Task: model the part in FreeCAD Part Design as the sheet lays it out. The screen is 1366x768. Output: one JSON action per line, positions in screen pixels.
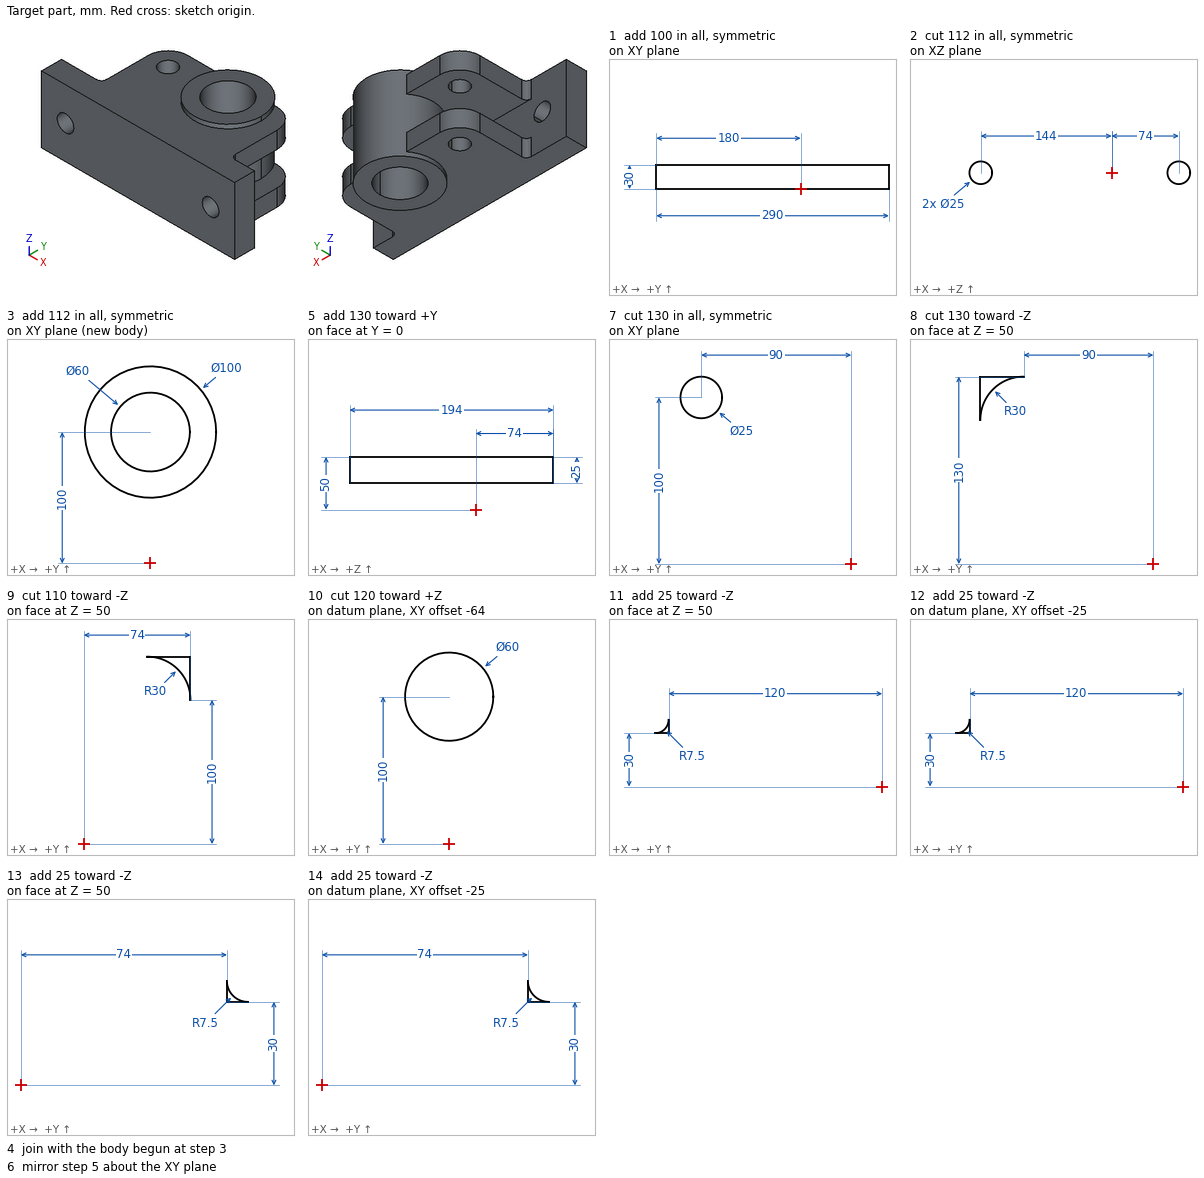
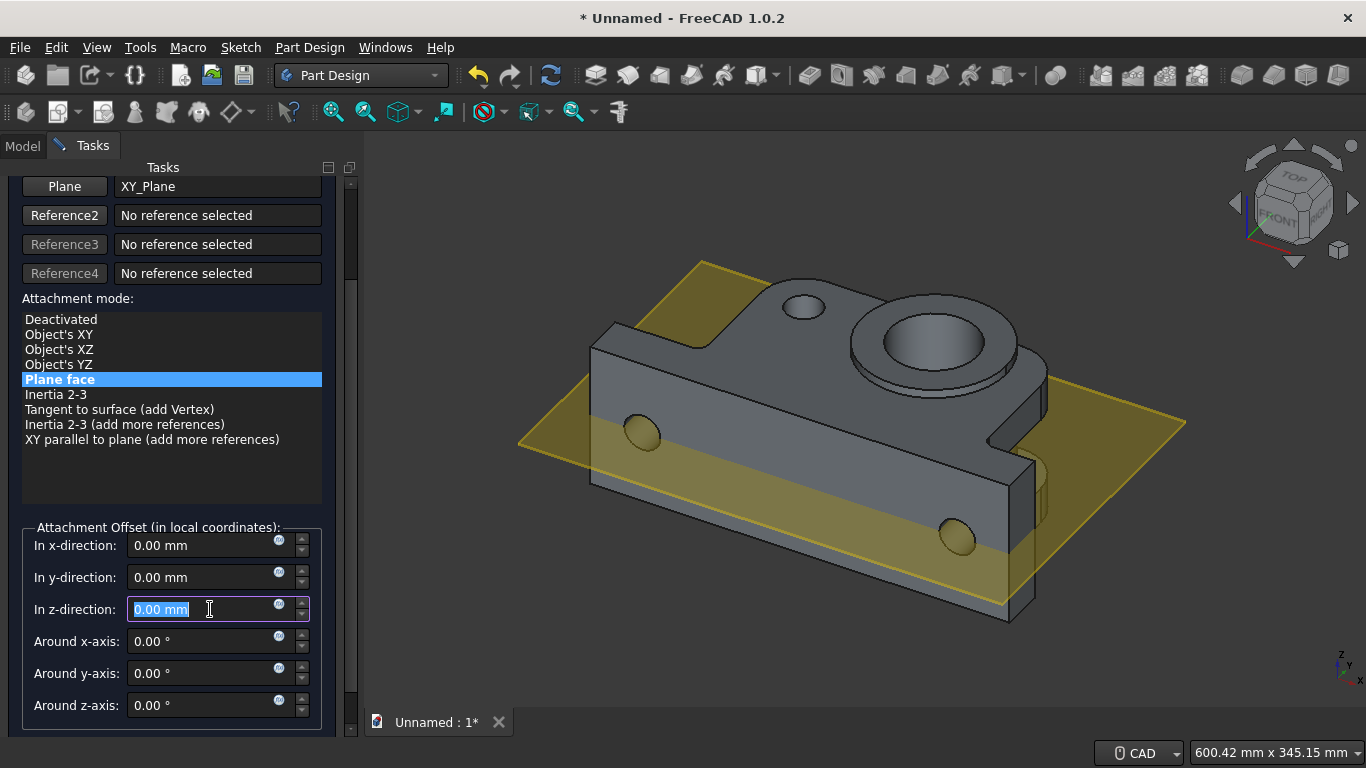
{"action": "type", "text": "-25"}
{"action": "key", "text": "Tab"}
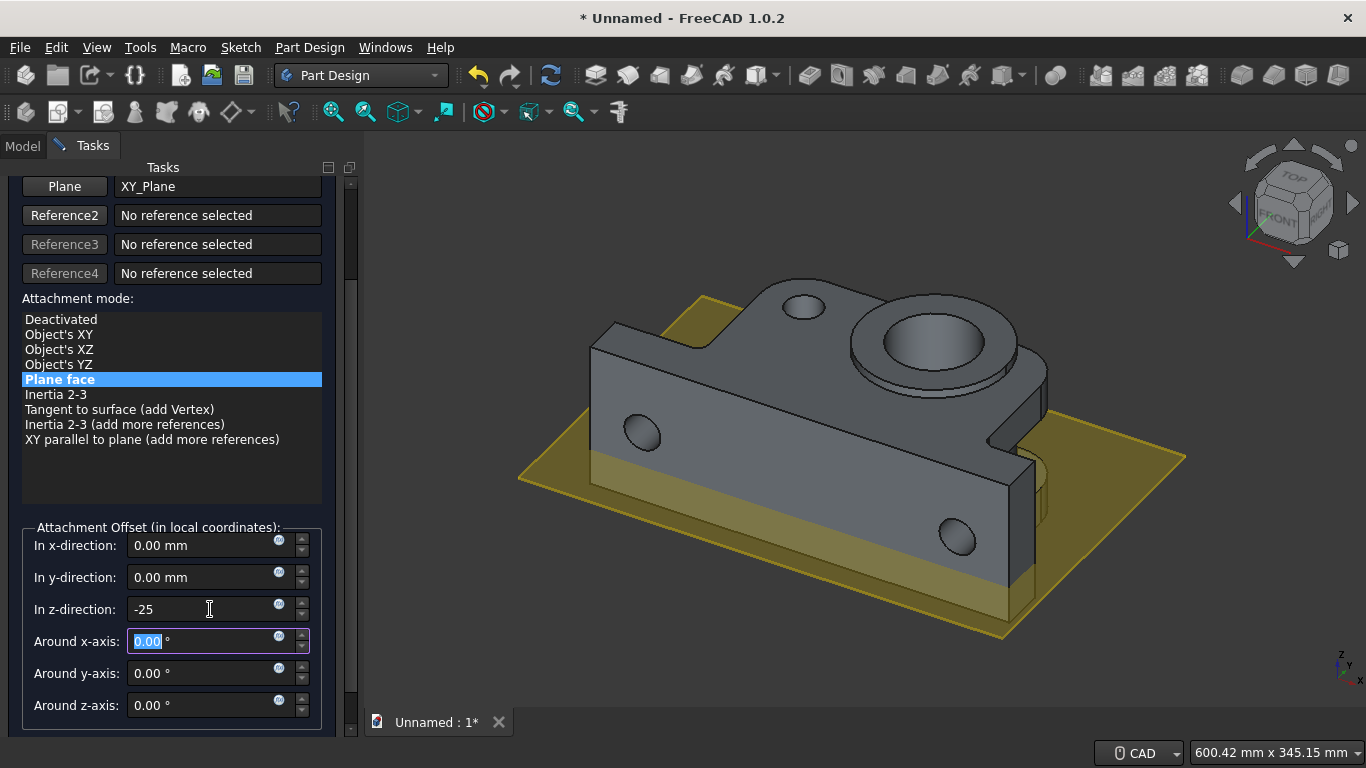
{"action": "scroll", "coordinate": [351, 456], "scroll_direction": "up", "scroll_amount": 3}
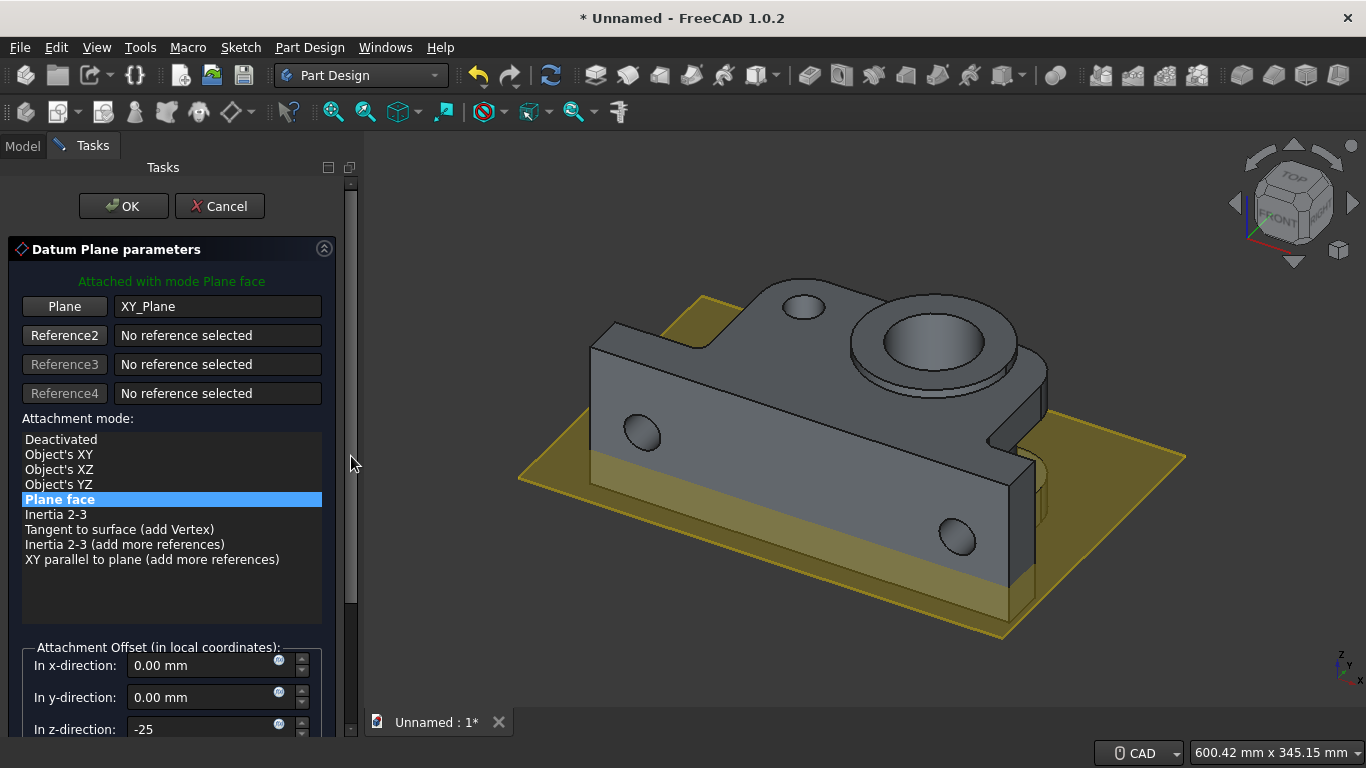
{"action": "left_click", "coordinate": [124, 206]}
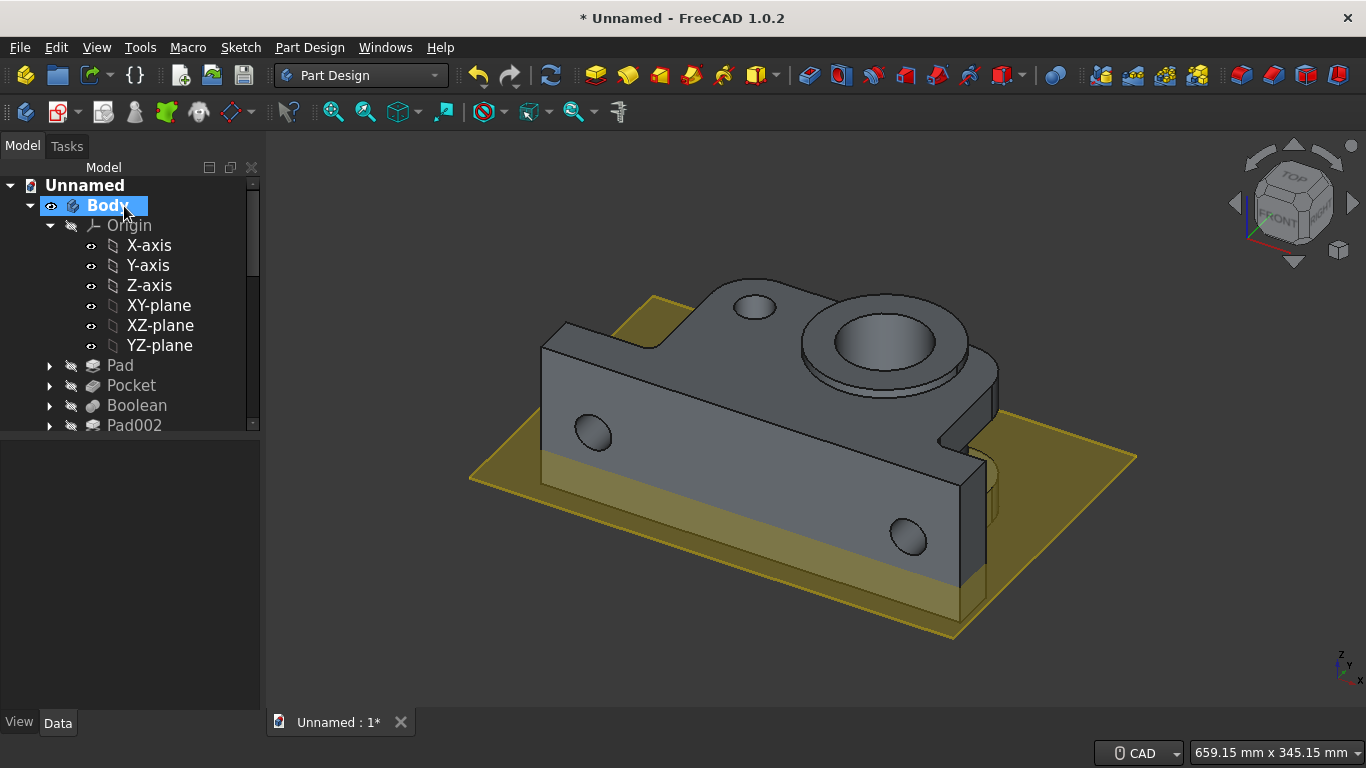
{"action": "scroll", "coordinate": [100, 301], "scroll_direction": "down", "scroll_amount": 3}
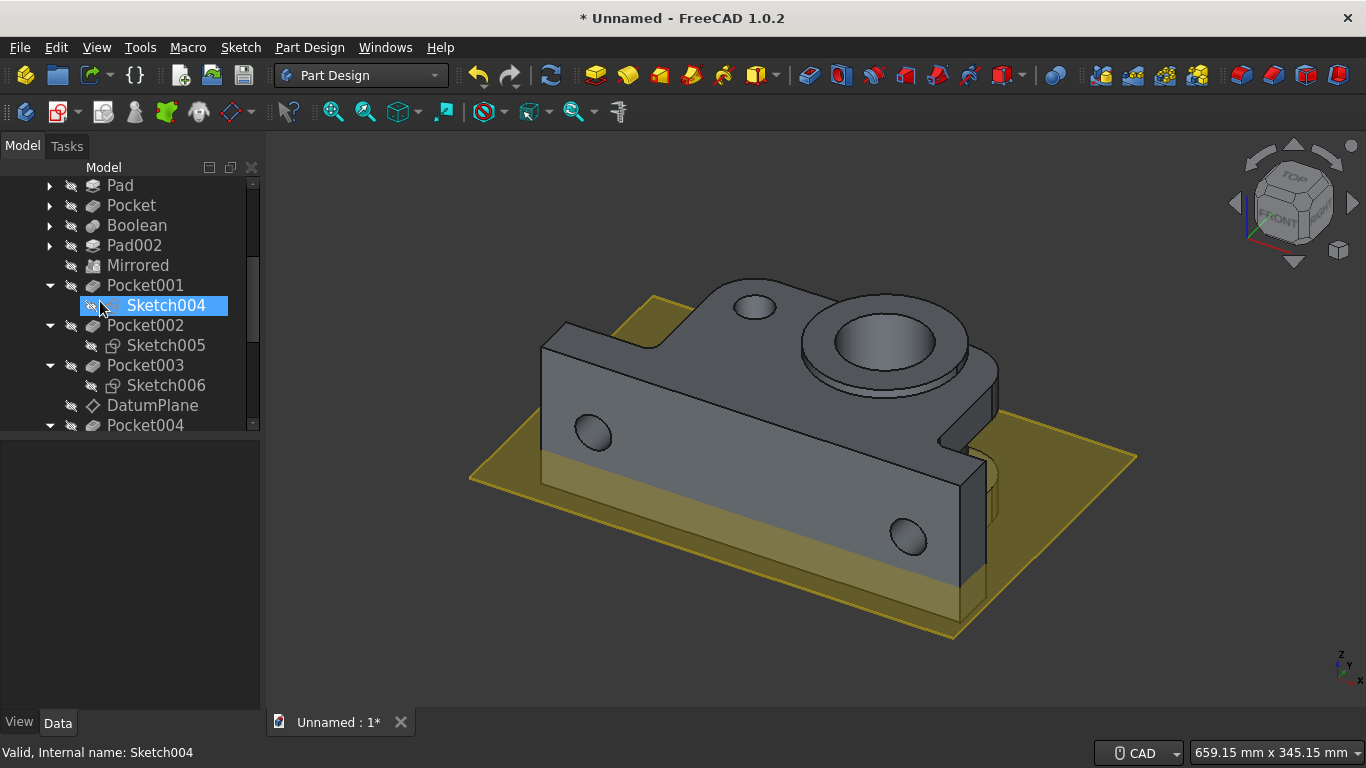
{"action": "scroll", "coordinate": [140, 301], "scroll_direction": "up", "scroll_amount": 15}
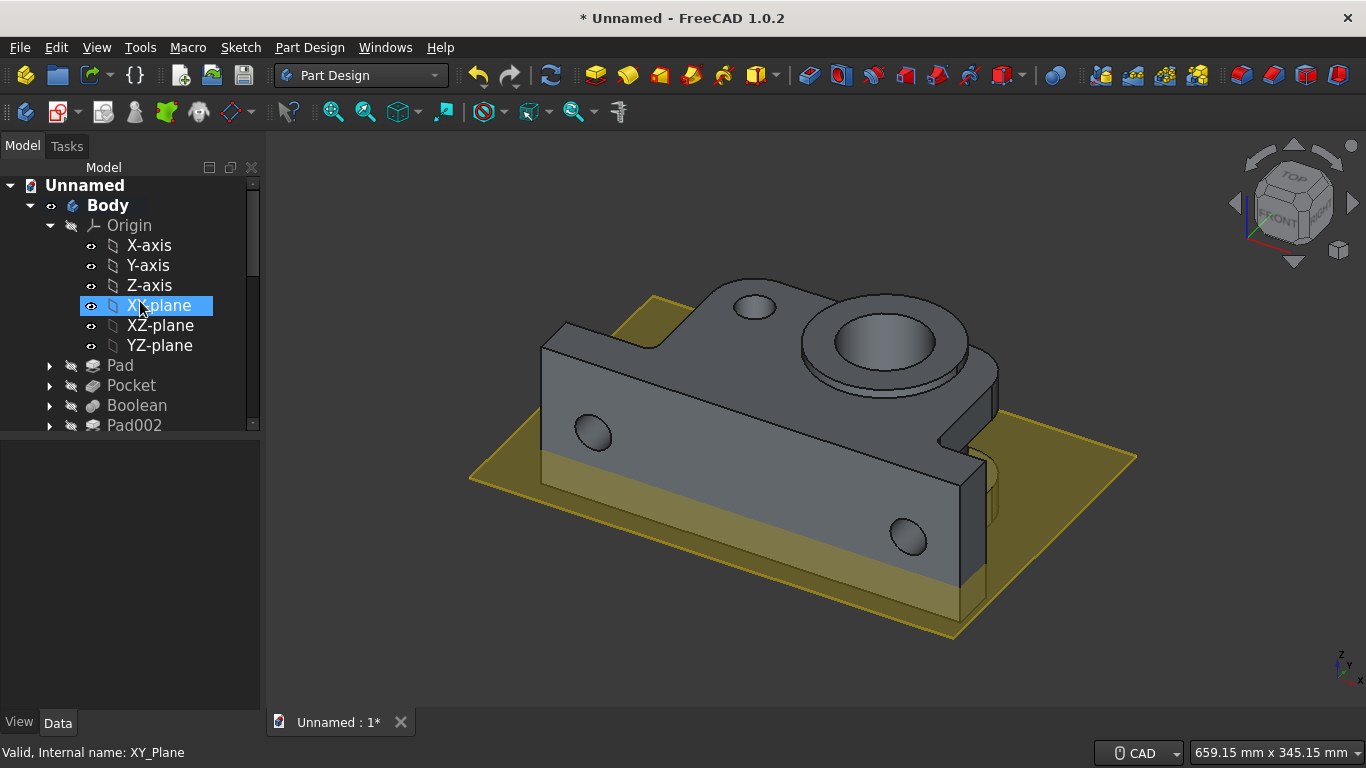
{"action": "scroll", "coordinate": [100, 301], "scroll_direction": "down", "scroll_amount": 6}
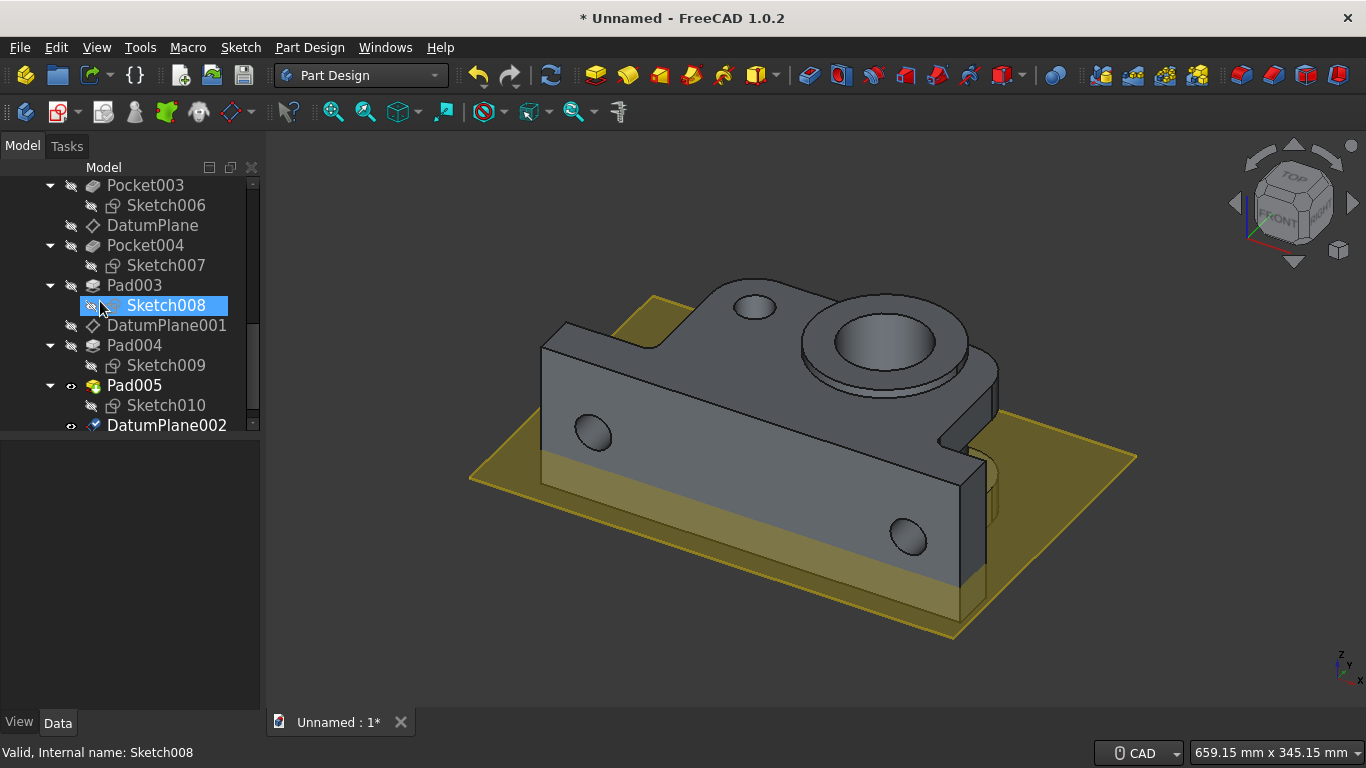
{"action": "left_click", "coordinate": [116, 426]}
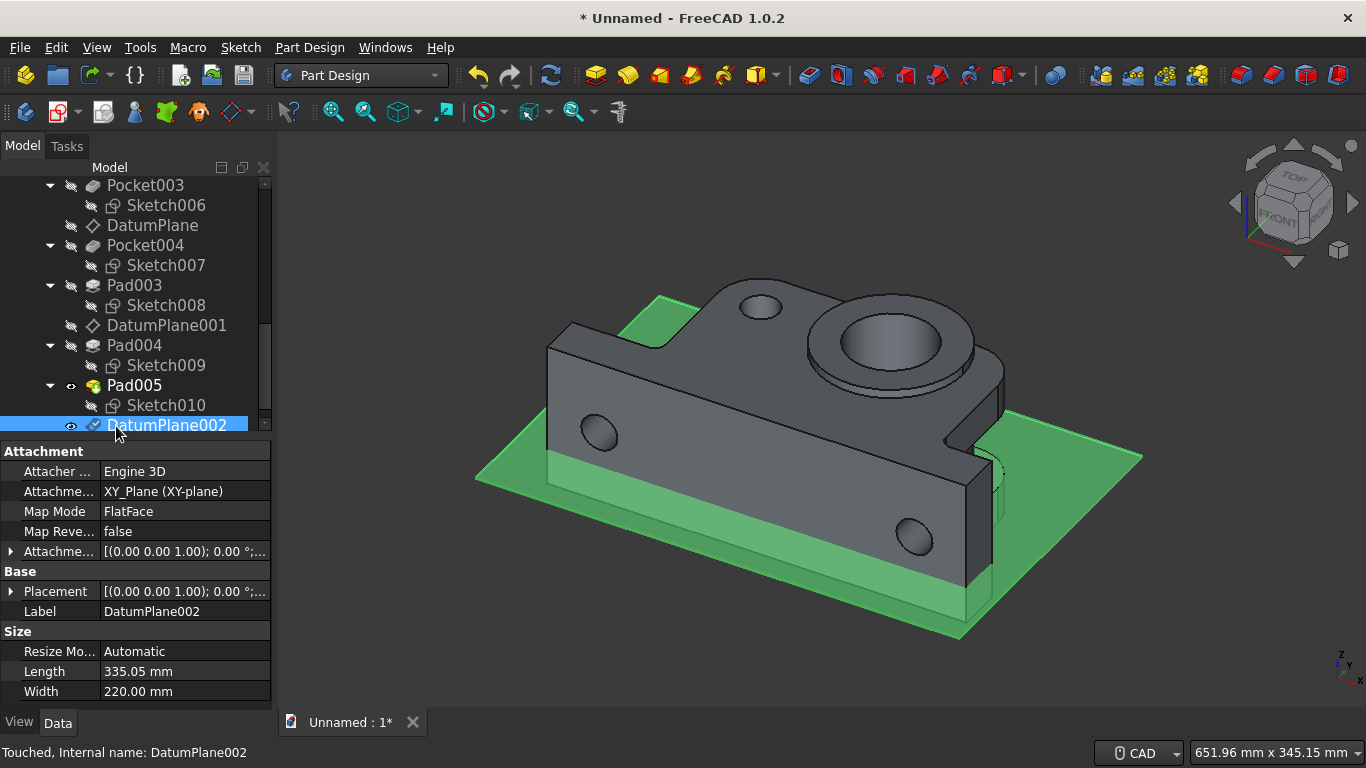
{"action": "left_click", "coordinate": [58, 112]}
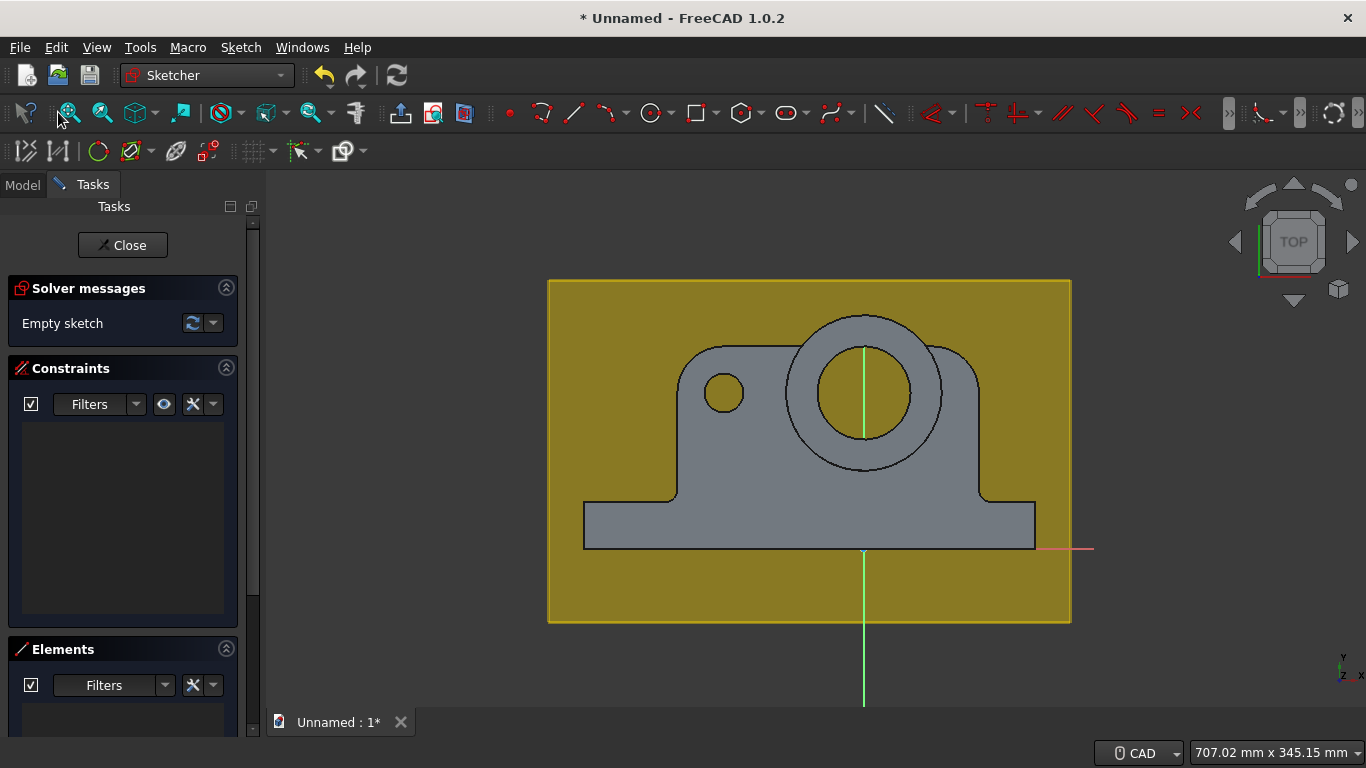
{"action": "left_click", "coordinate": [466, 114]}